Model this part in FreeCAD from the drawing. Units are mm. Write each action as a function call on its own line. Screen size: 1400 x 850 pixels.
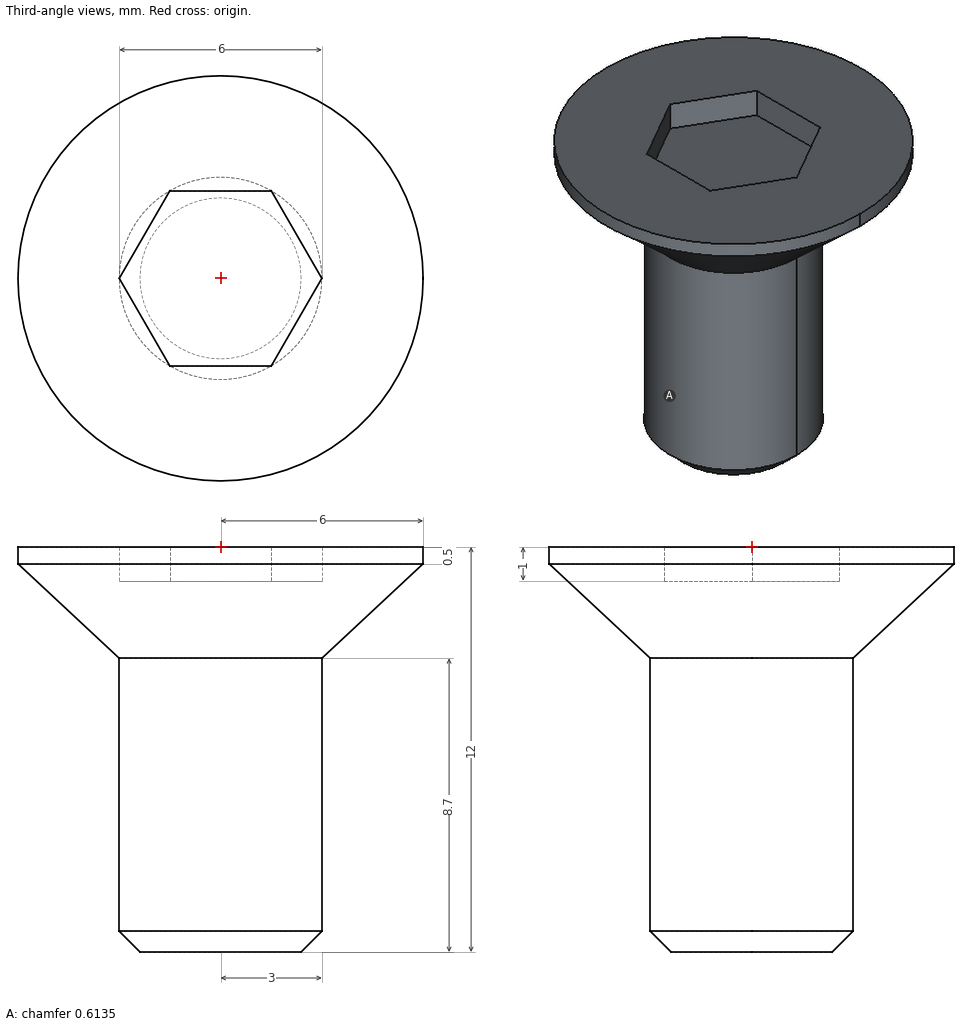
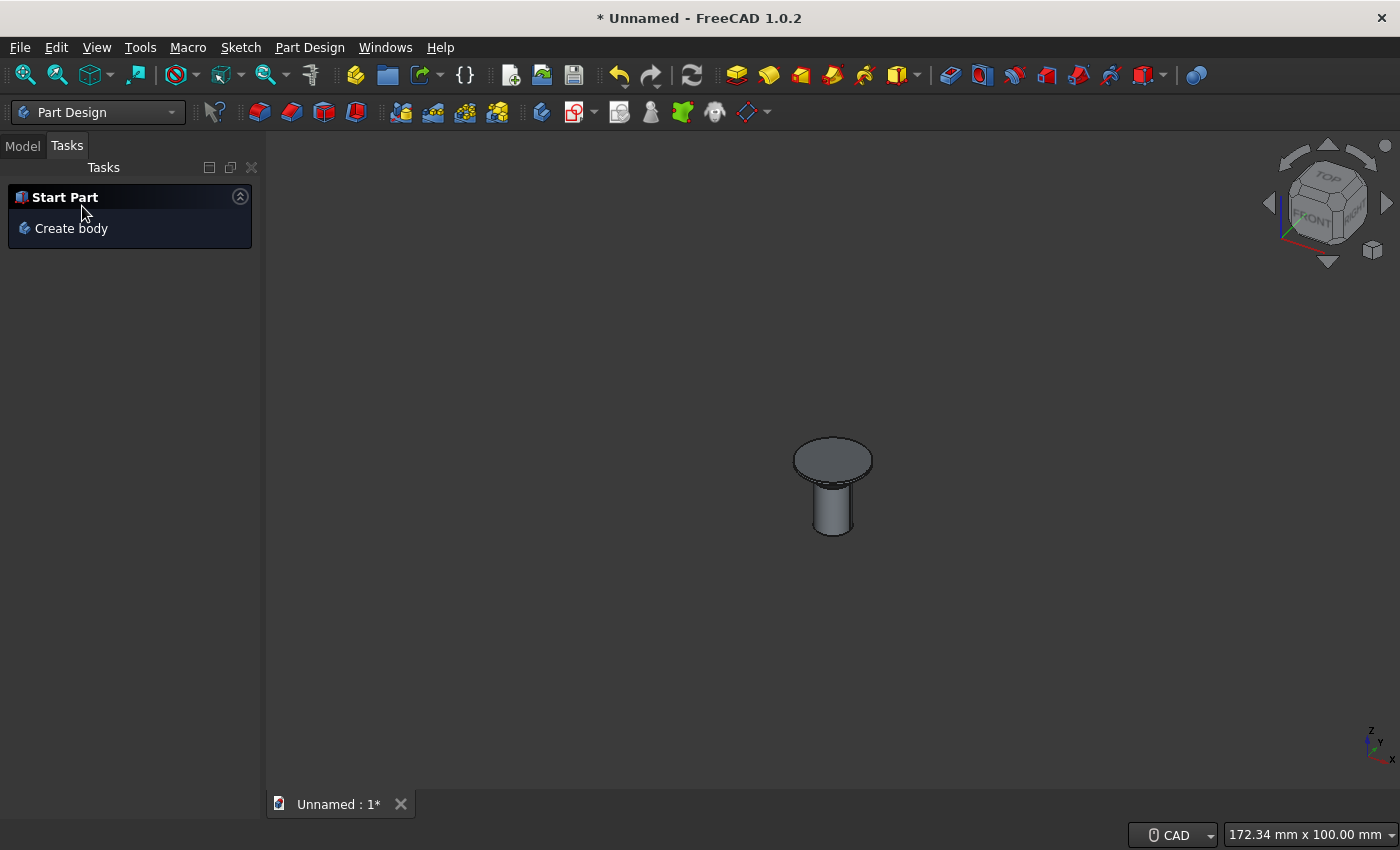
key(v)
key(f)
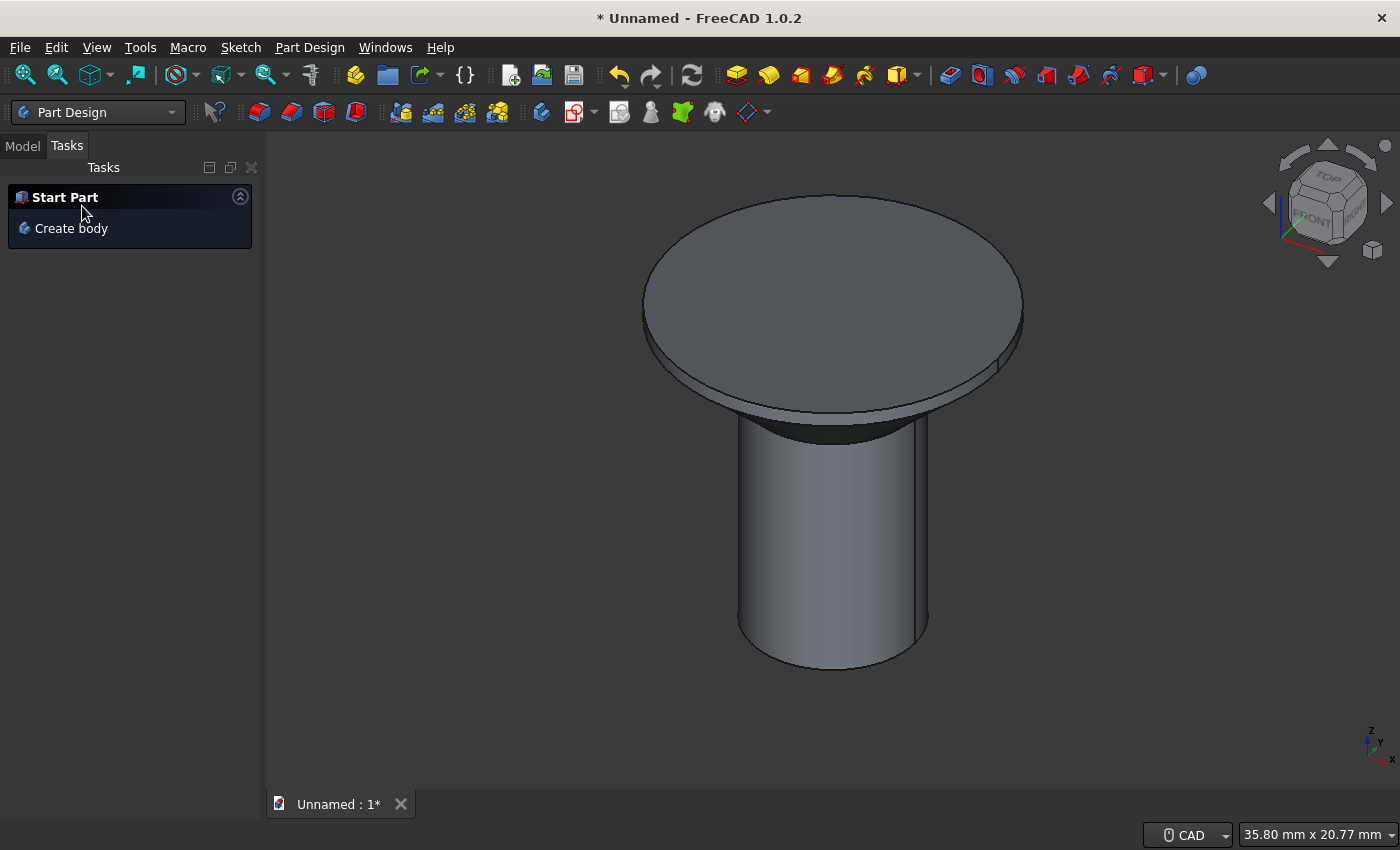
click(833, 303)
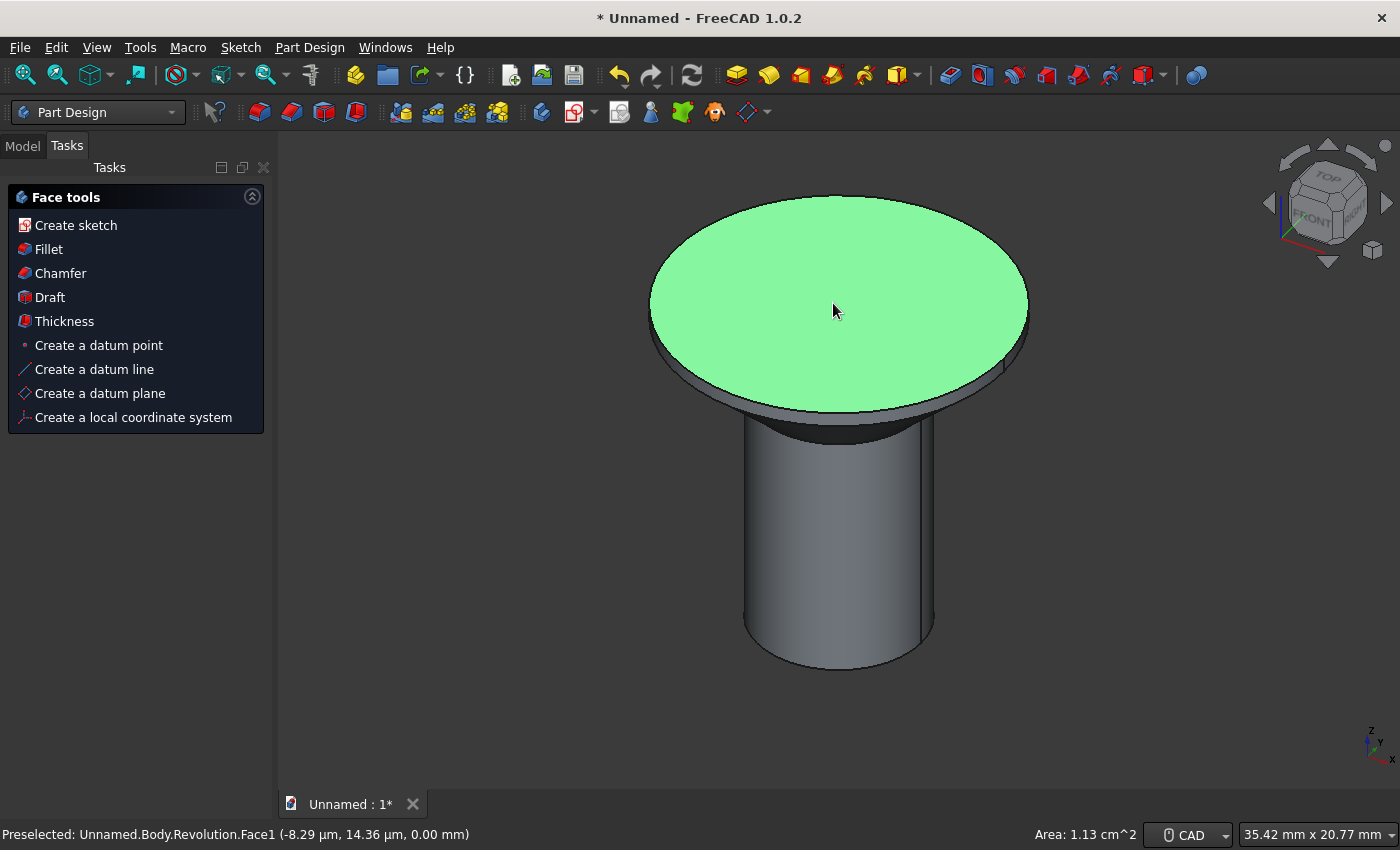
click(574, 112)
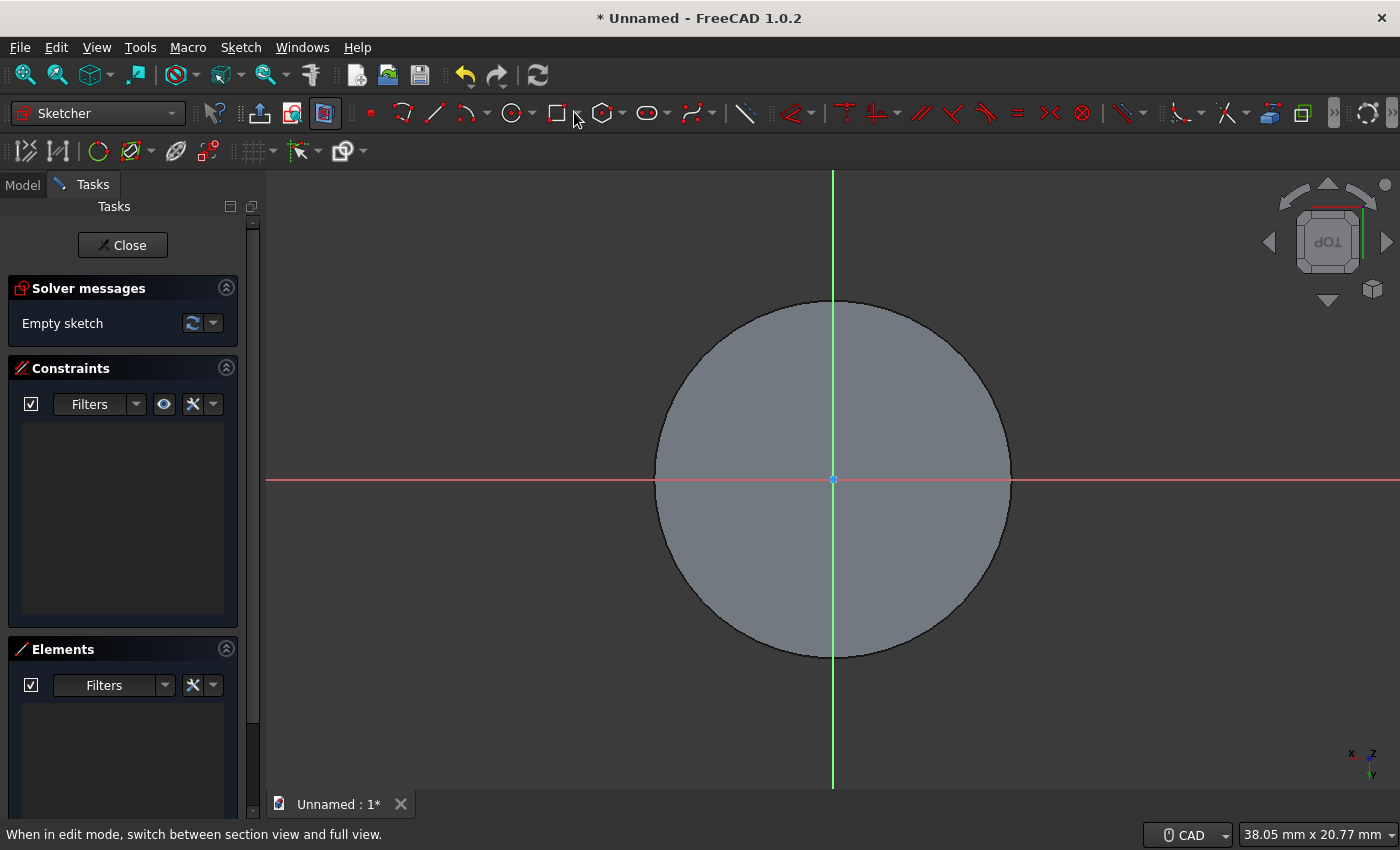
scroll(873, 479, up, 5)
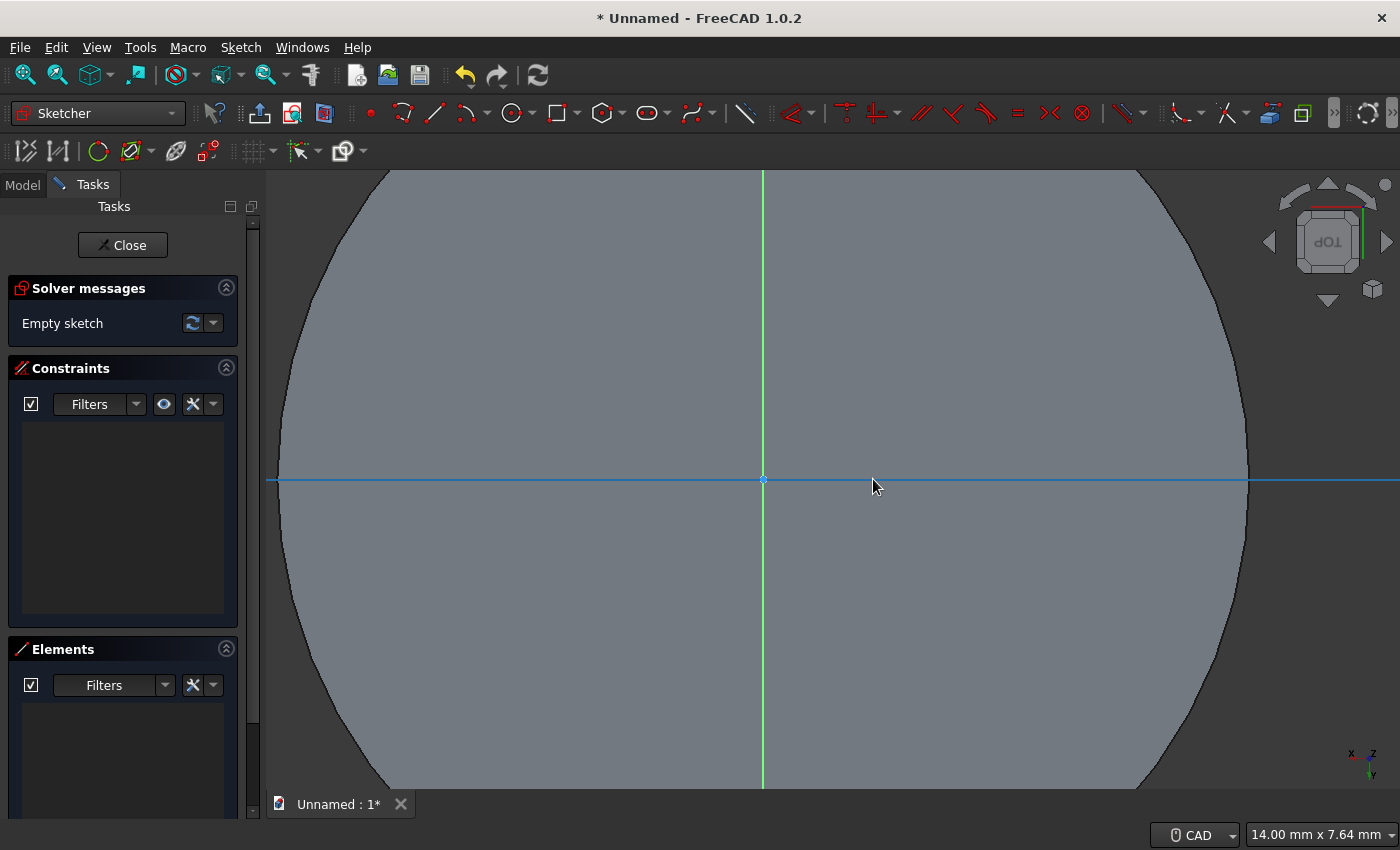
key(g)
key(p)
key(6)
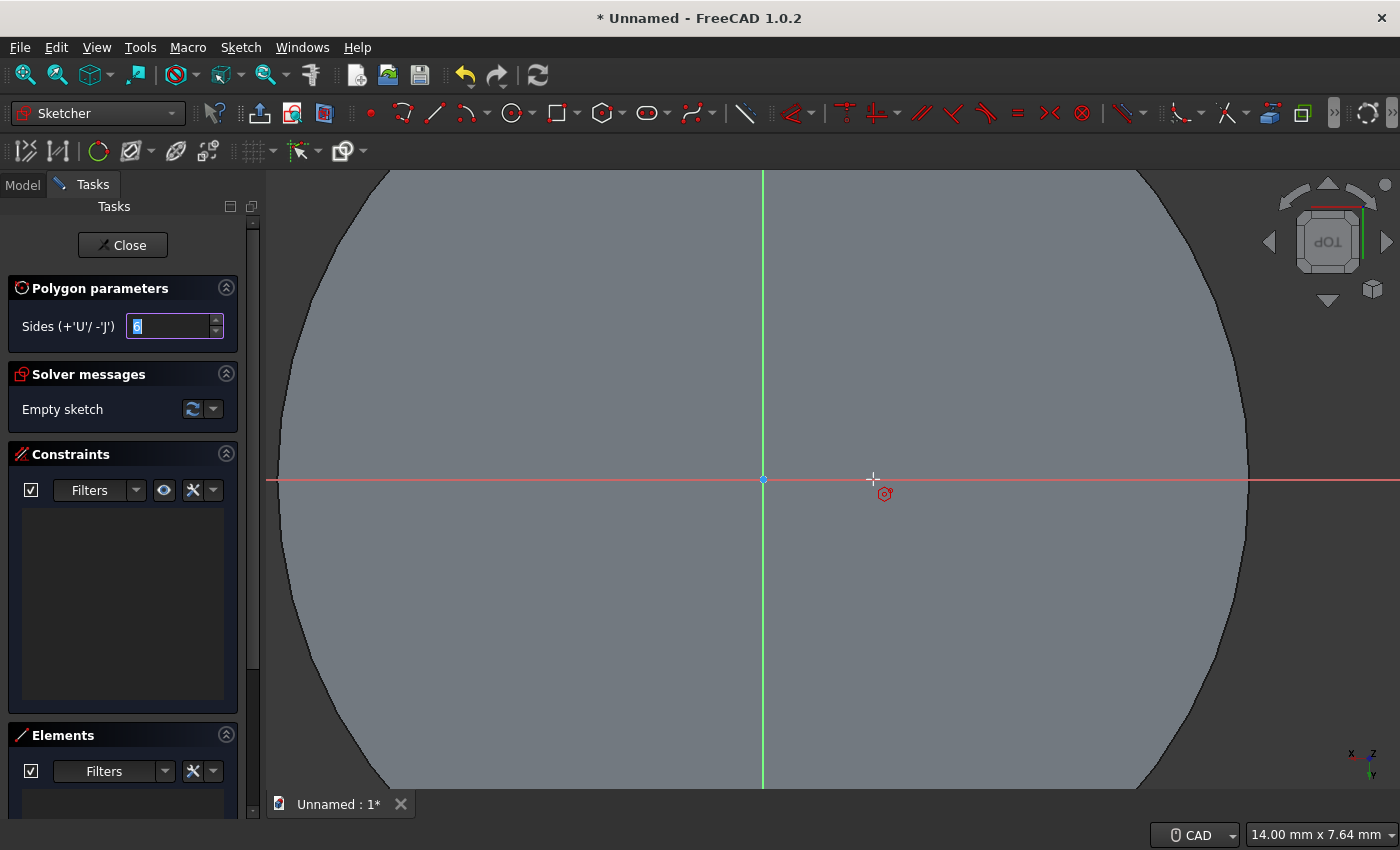
click(763, 479)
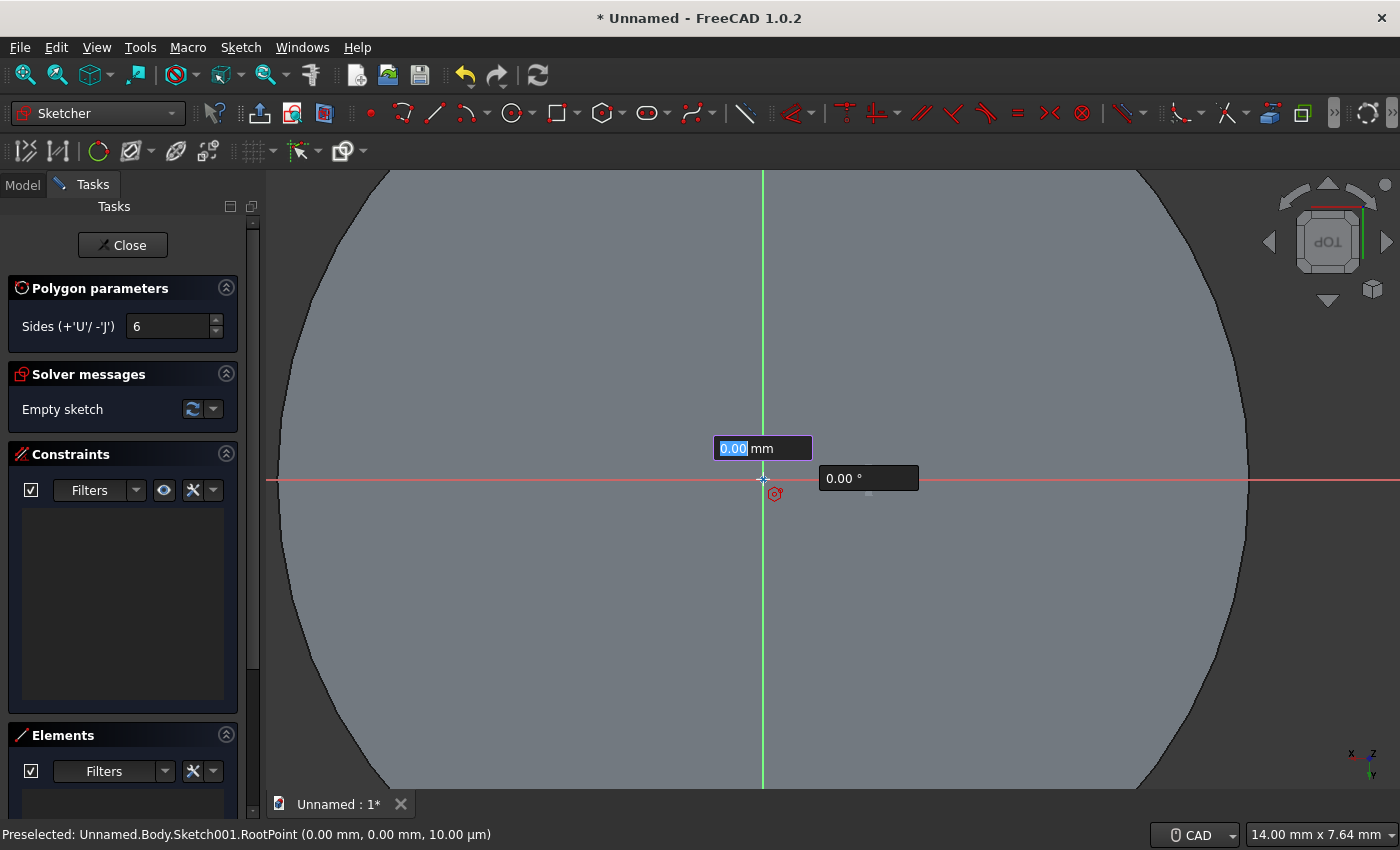
click(520, 479)
right_click(520, 479)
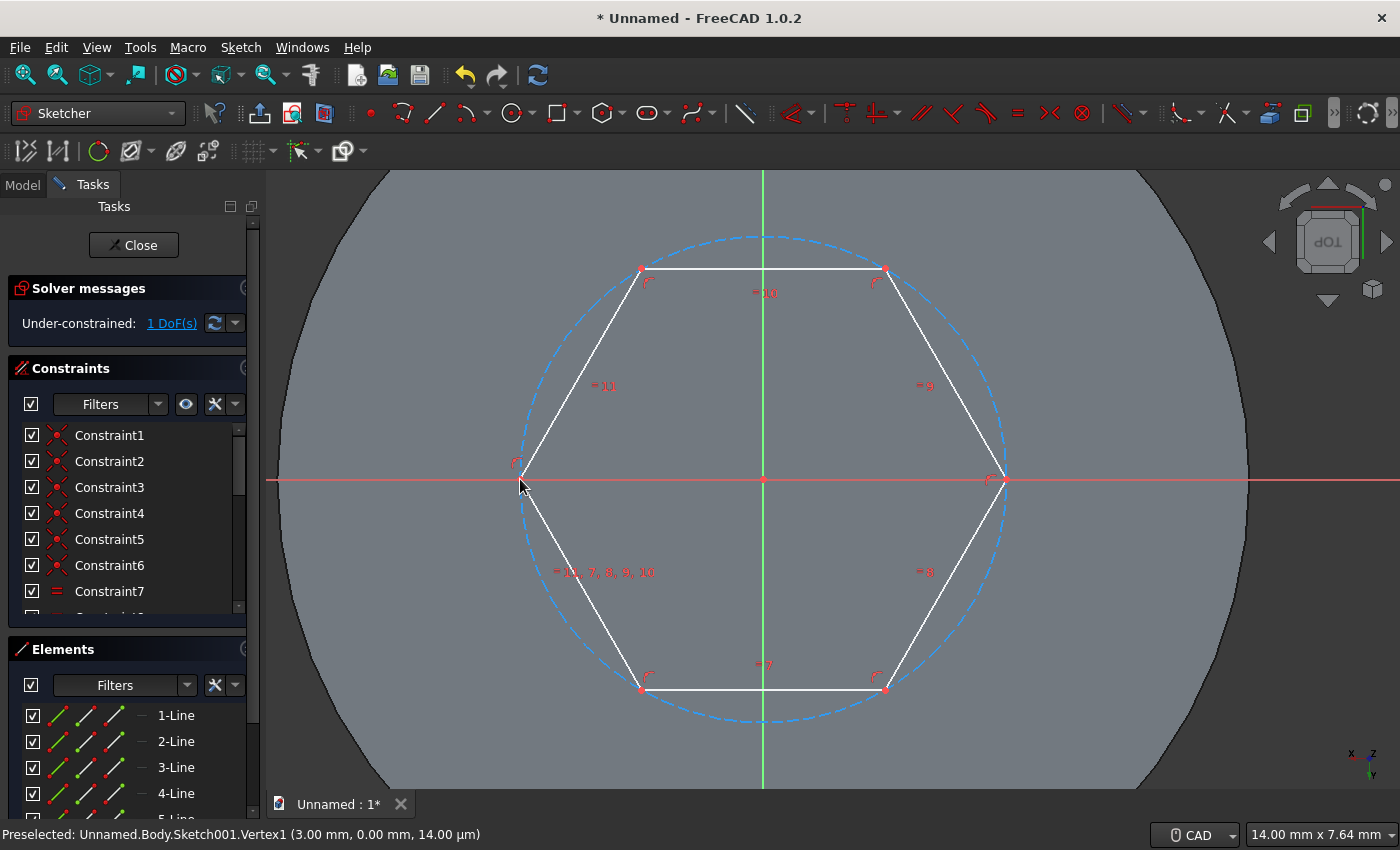
key(d)